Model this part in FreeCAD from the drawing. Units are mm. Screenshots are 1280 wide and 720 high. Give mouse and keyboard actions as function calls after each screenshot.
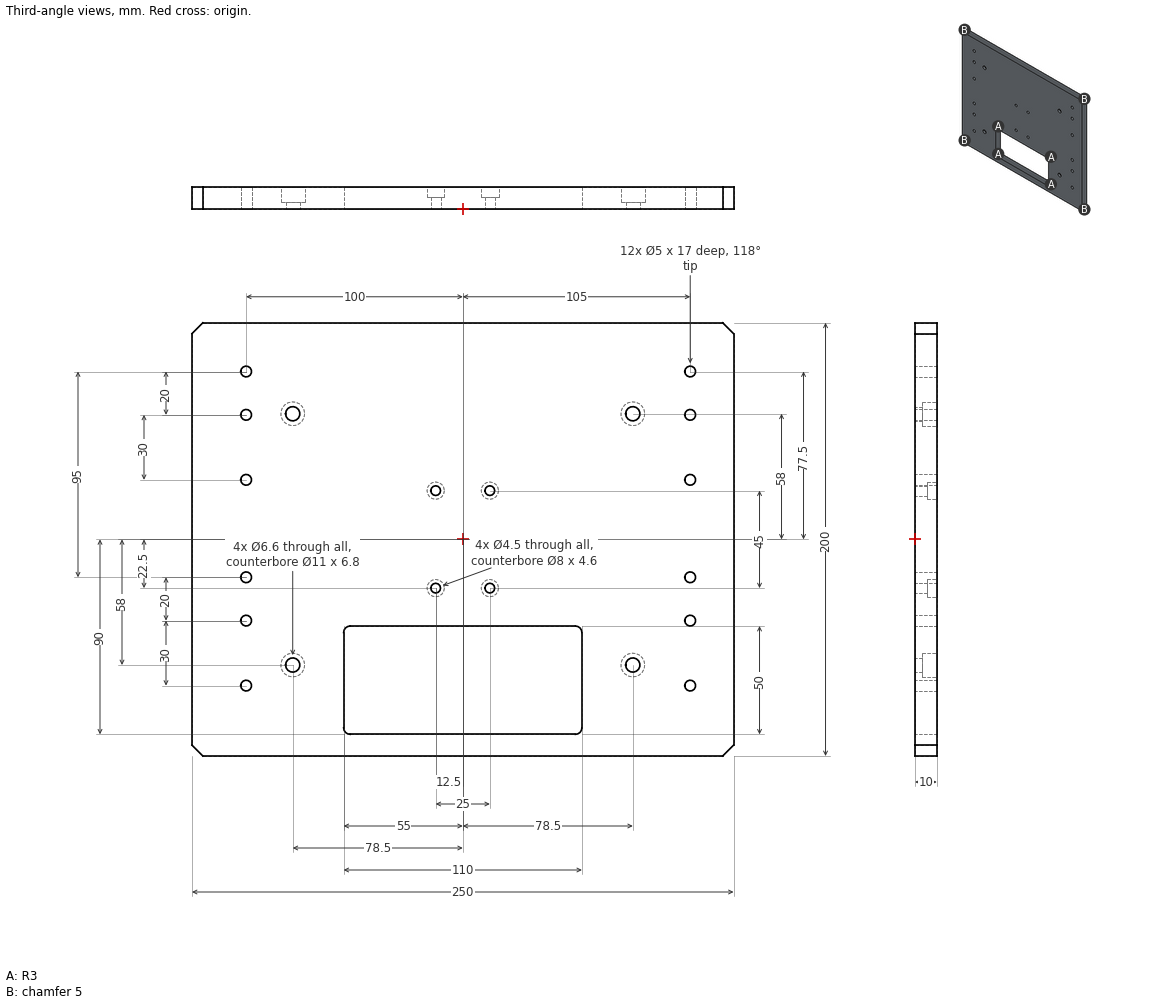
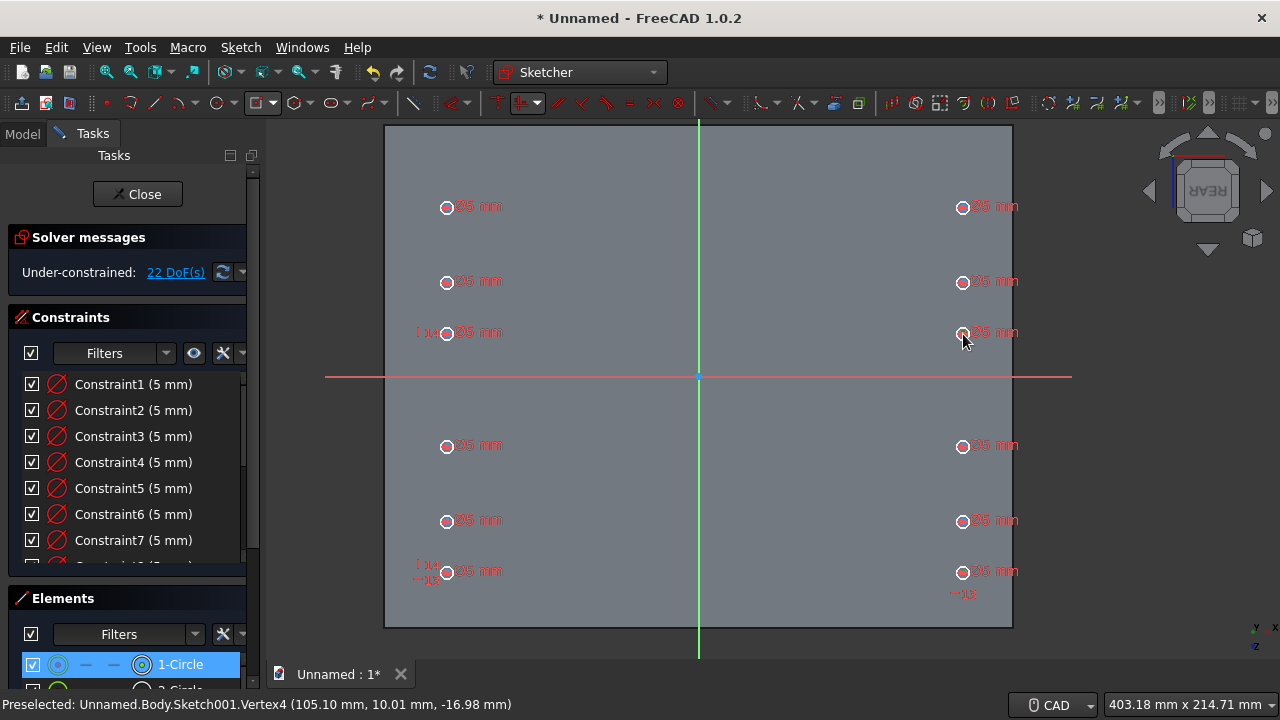
click(540, 104)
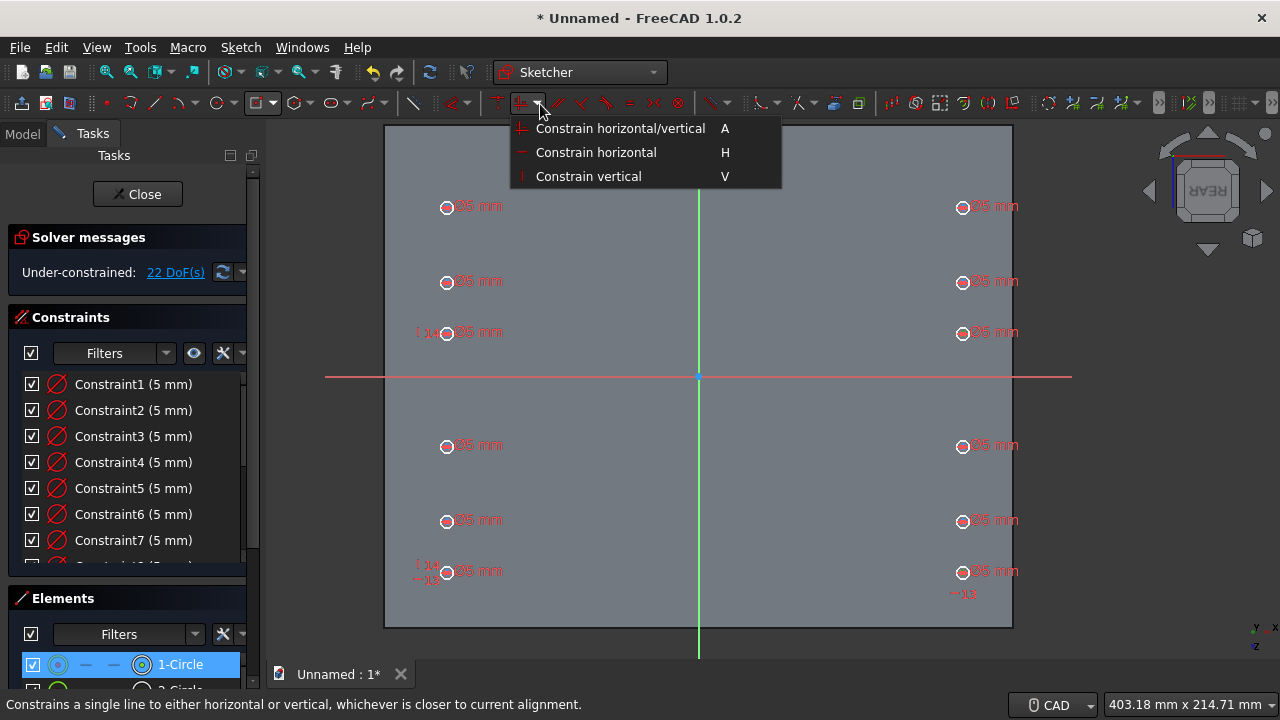
click(646, 176)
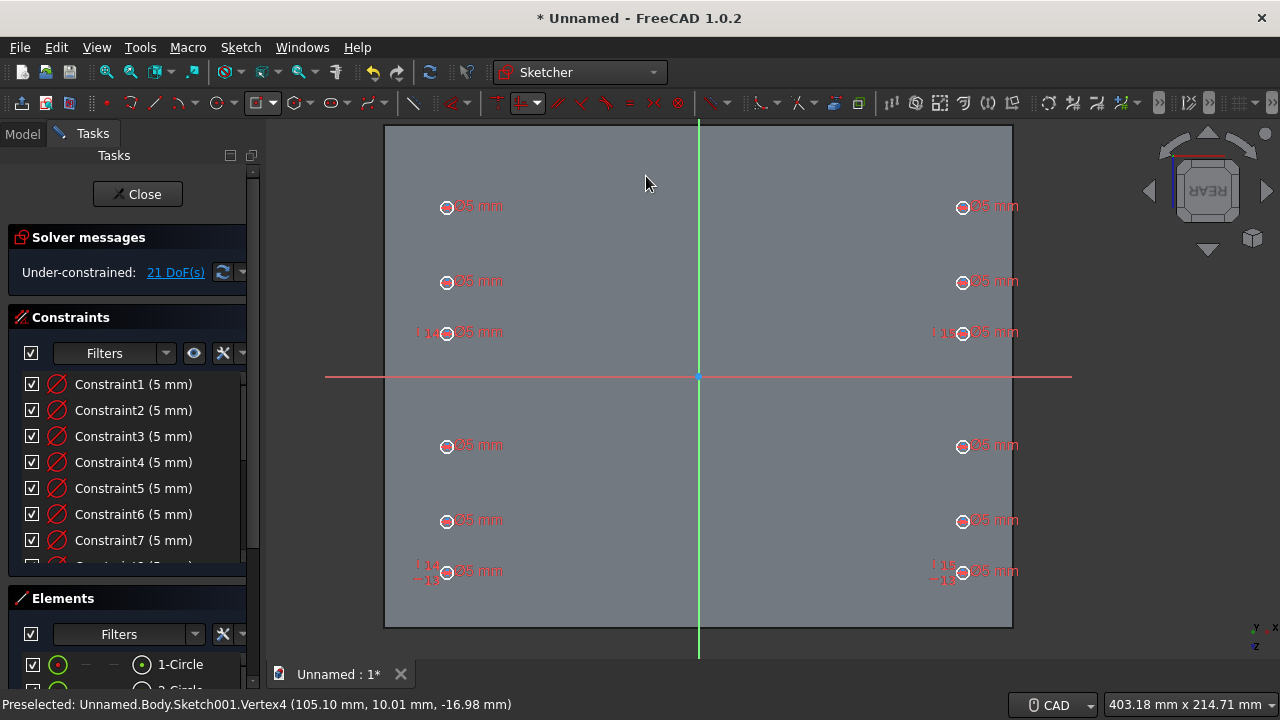
click(447, 334)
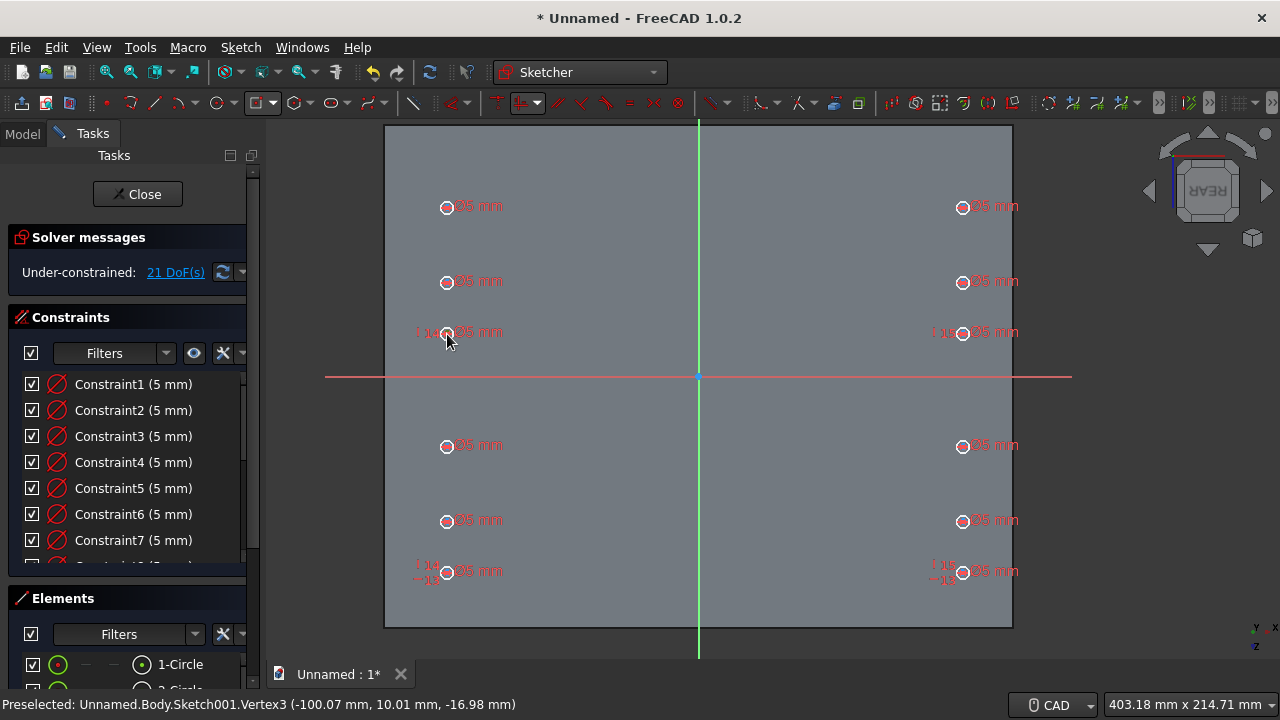
click(963, 334)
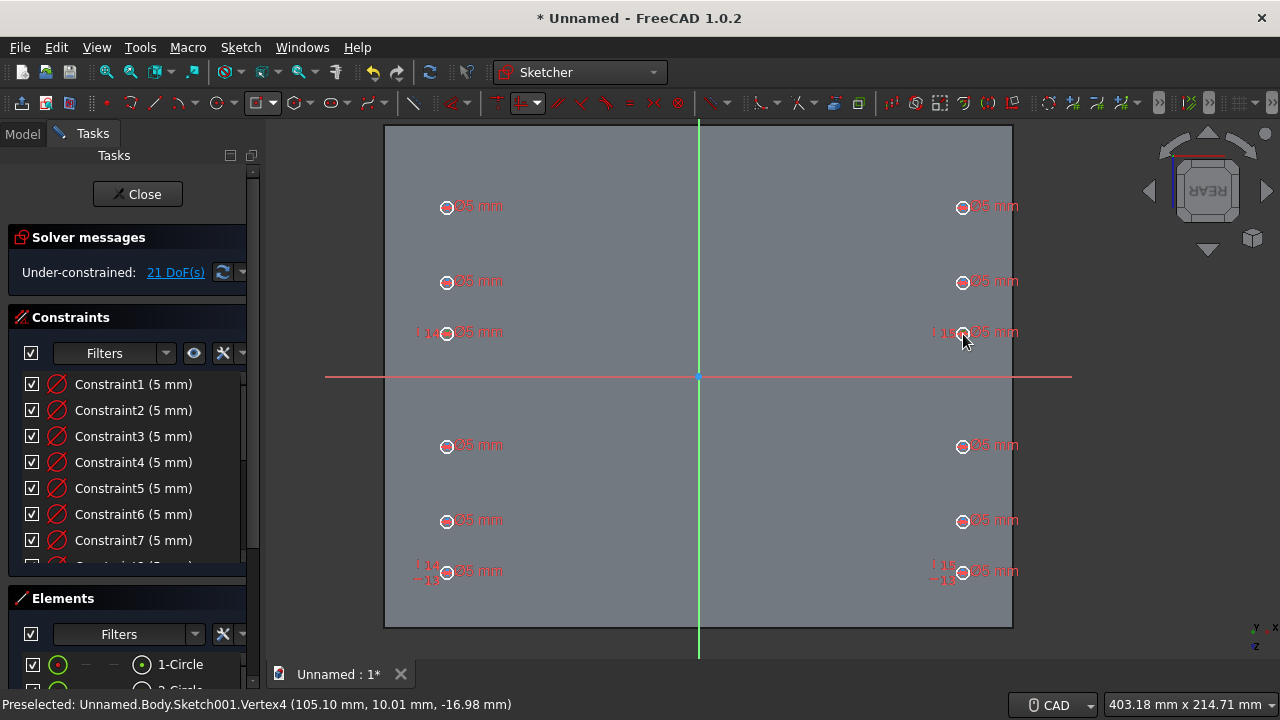
click(540, 104)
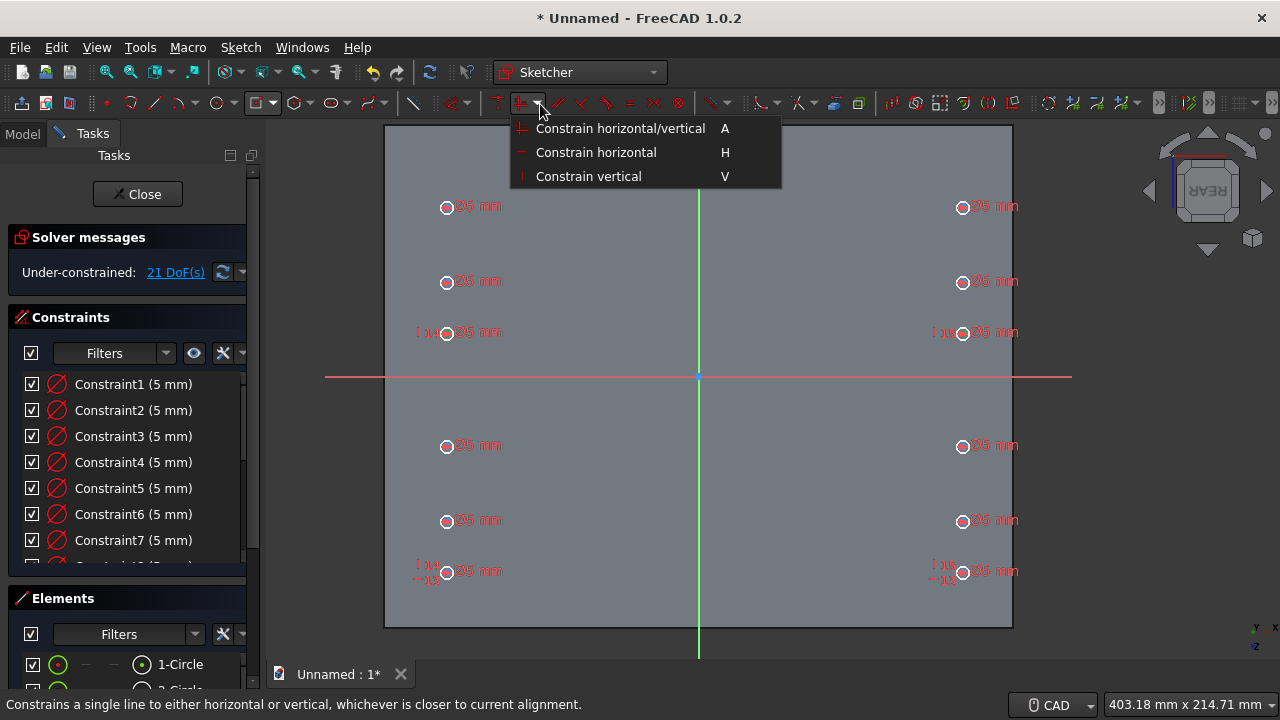
click(646, 152)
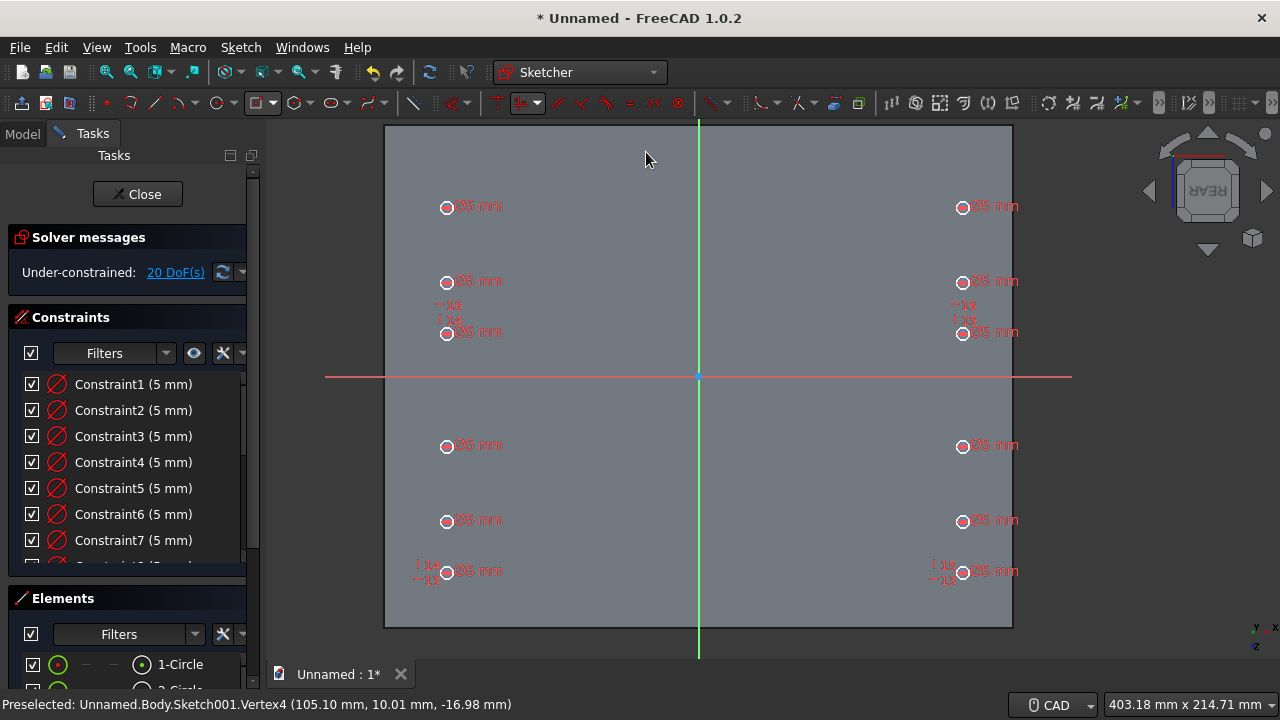
click(447, 334)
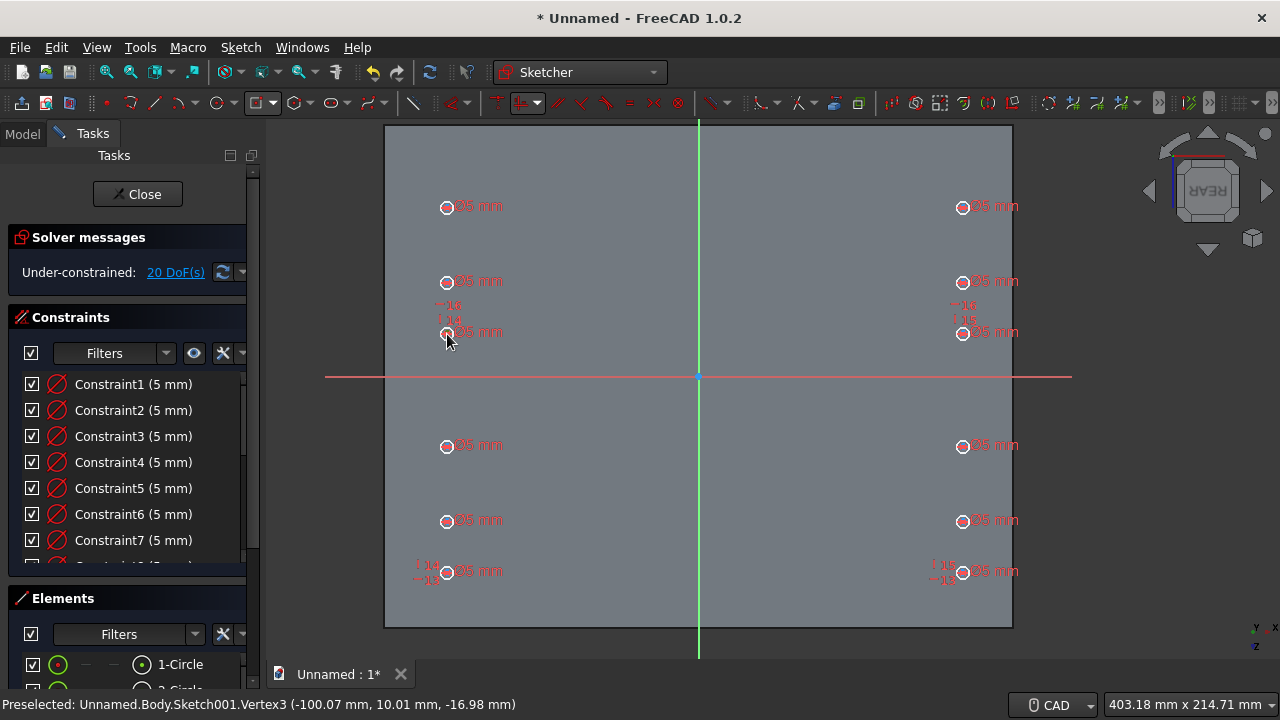
click(447, 283)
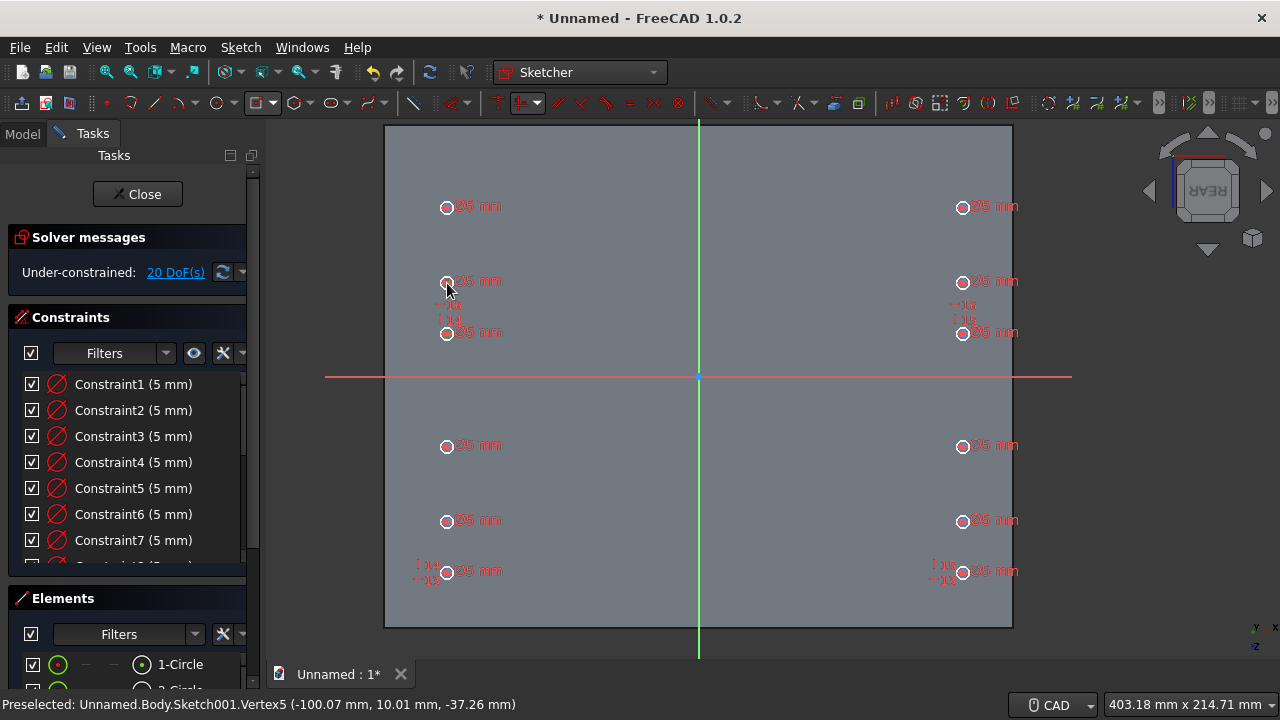
click(540, 104)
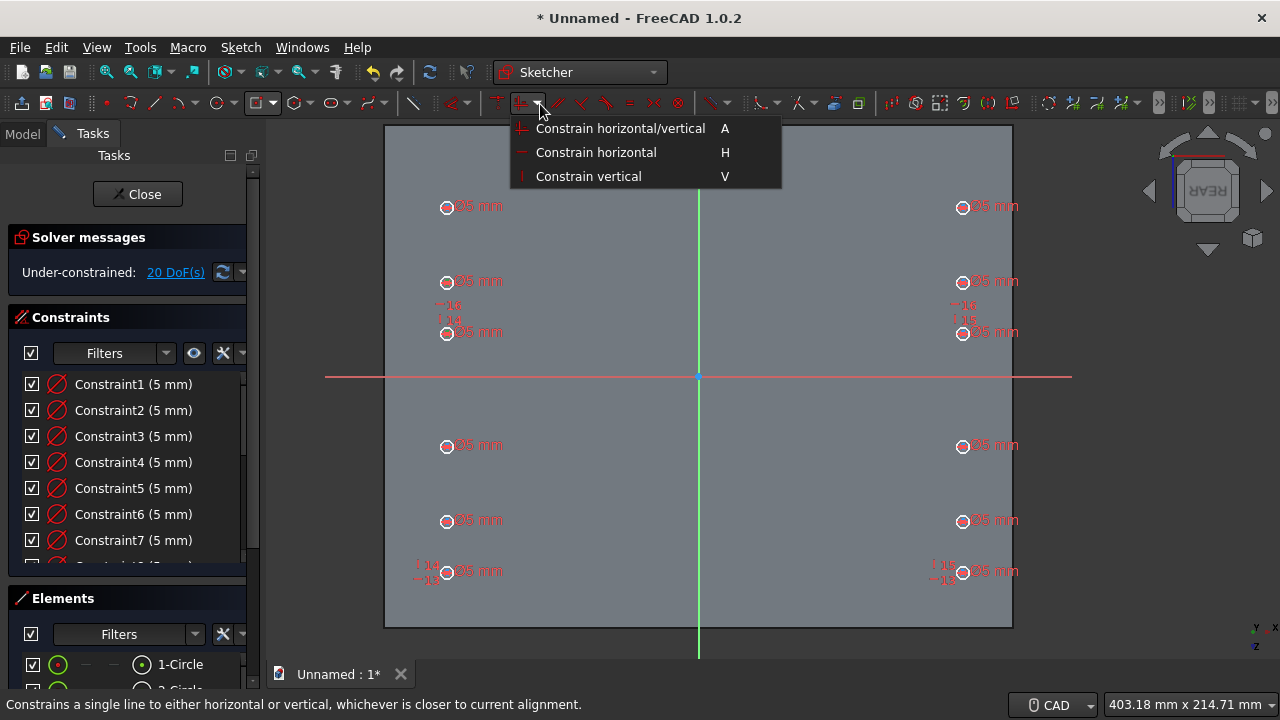
click(646, 176)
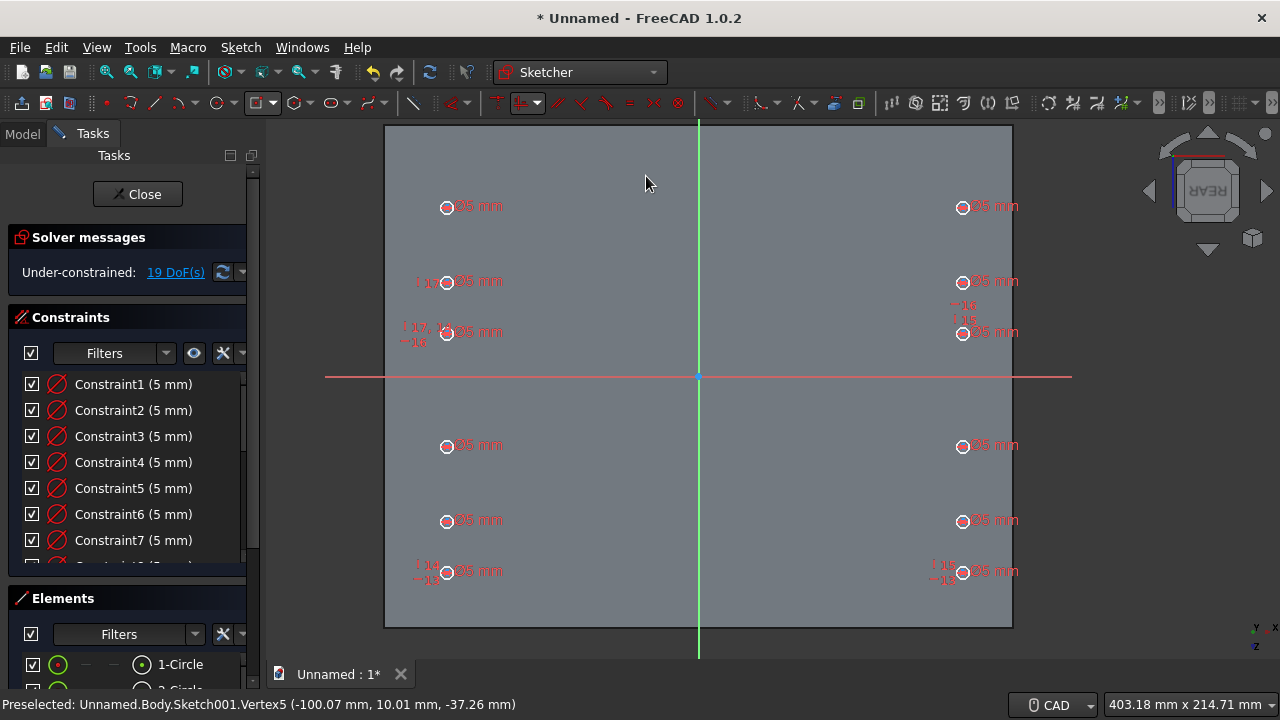
click(447, 283)